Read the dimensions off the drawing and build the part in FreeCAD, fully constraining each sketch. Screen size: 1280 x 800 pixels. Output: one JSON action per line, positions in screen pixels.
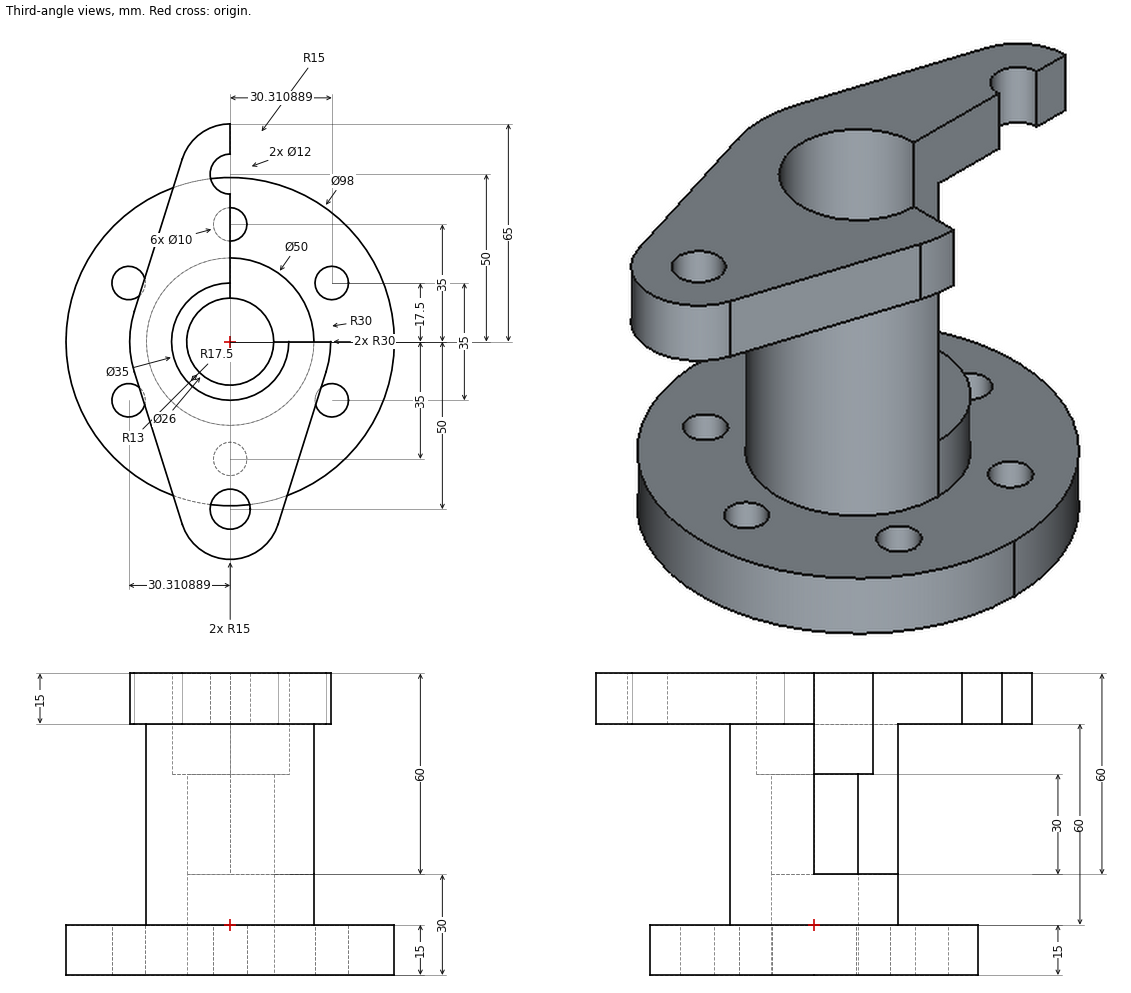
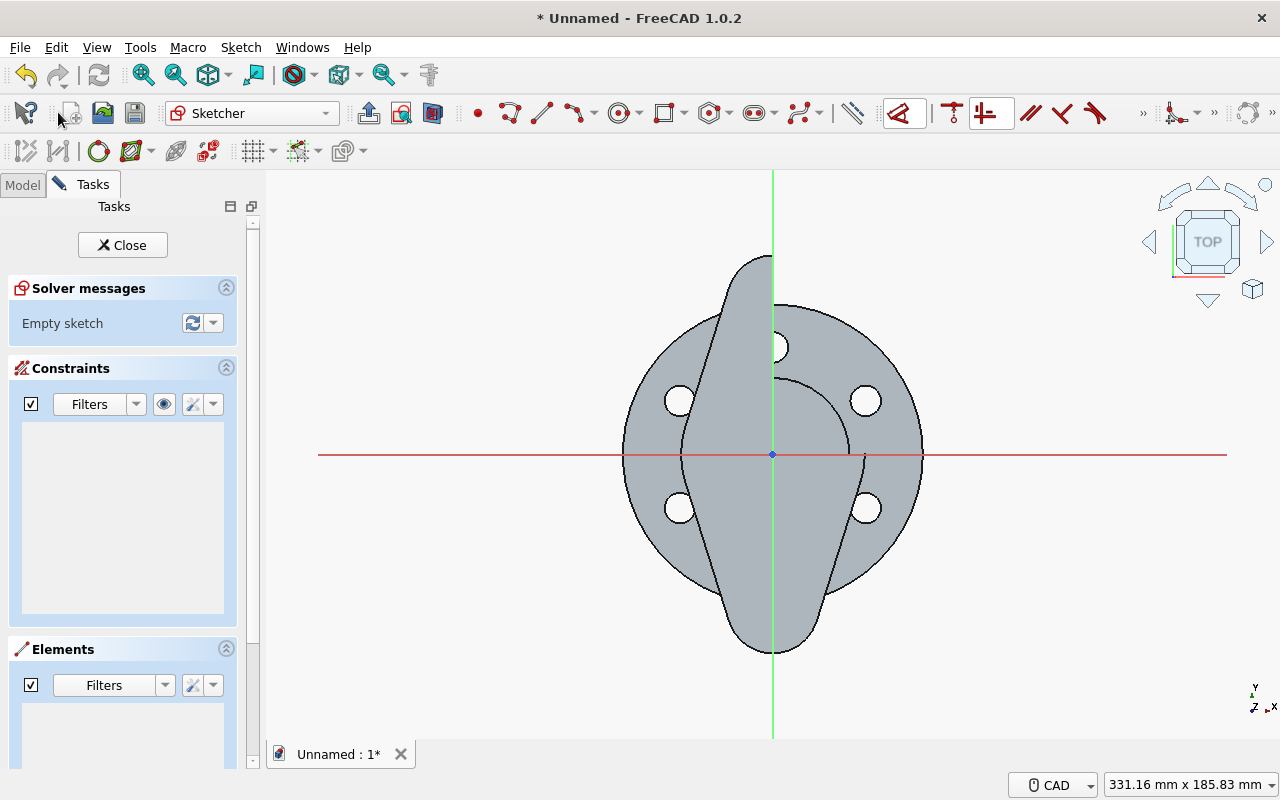
{"action": "key", "text": "g c"}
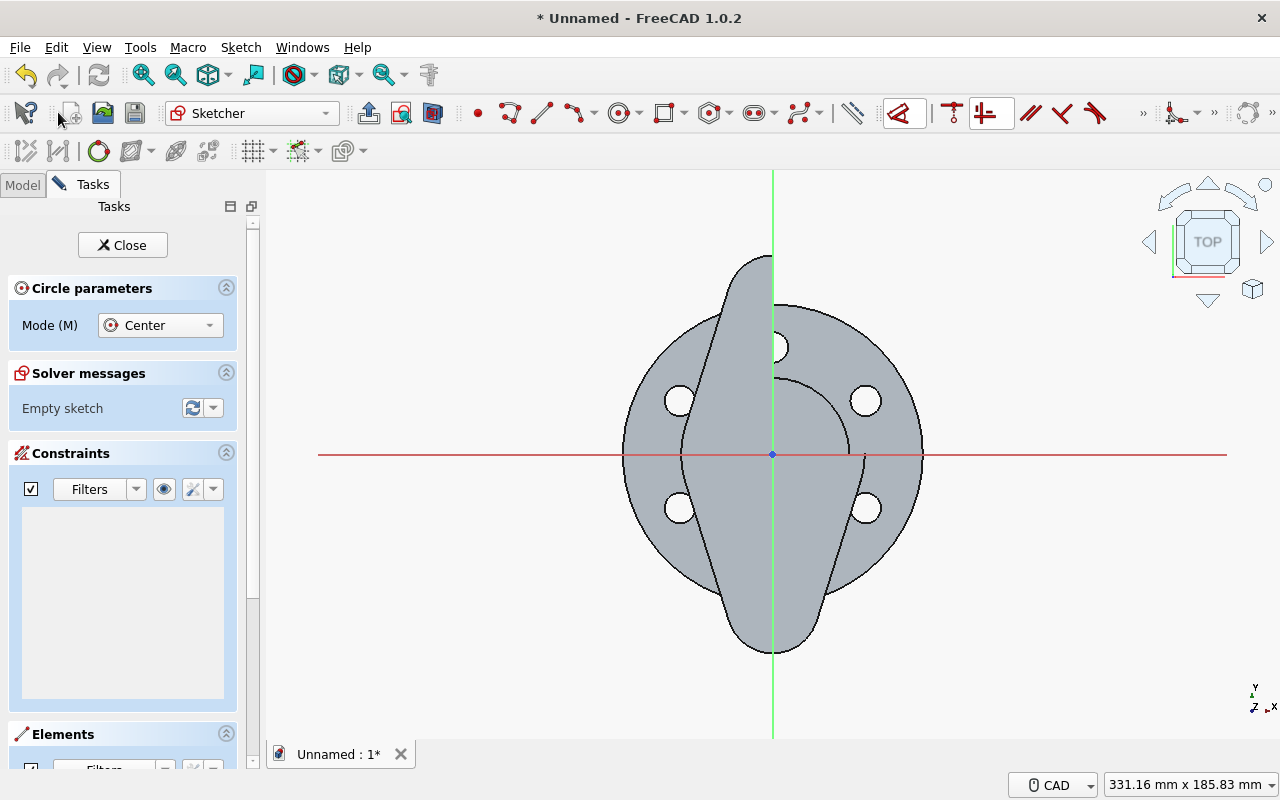
{"action": "left_click", "coordinate": [773, 454]}
{"action": "left_click", "coordinate": [811, 417]}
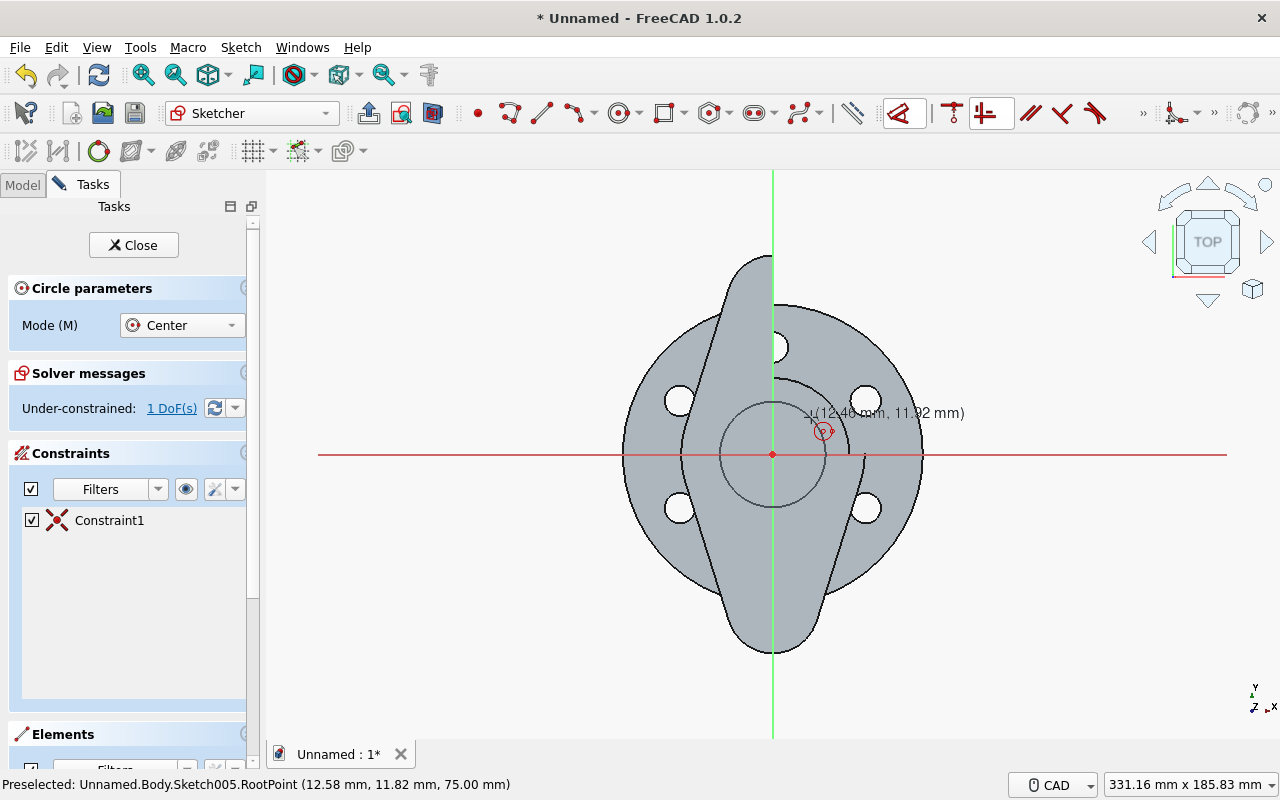
{"action": "scroll", "coordinate": [773, 301], "scroll_direction": "up", "scroll_amount": 2}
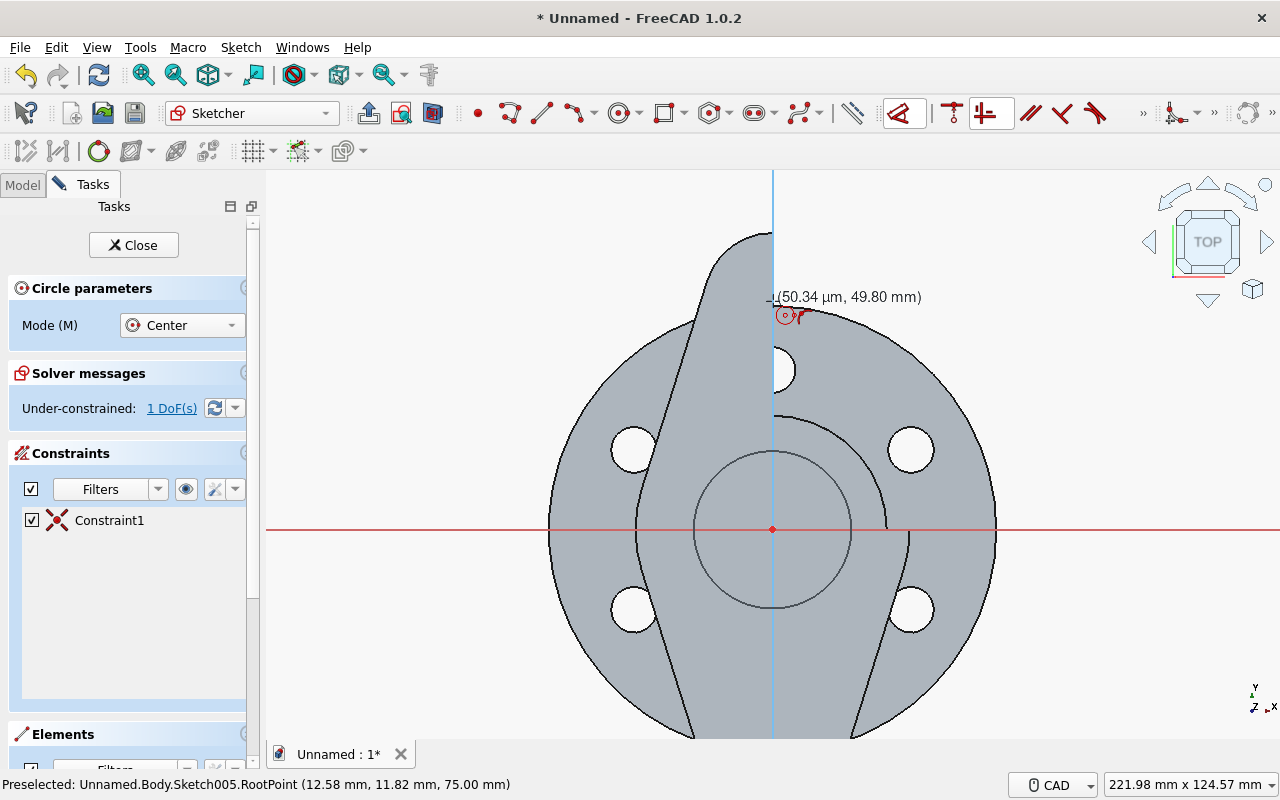
{"action": "left_click", "coordinate": [773, 301]}
{"action": "left_click", "coordinate": [792, 282]}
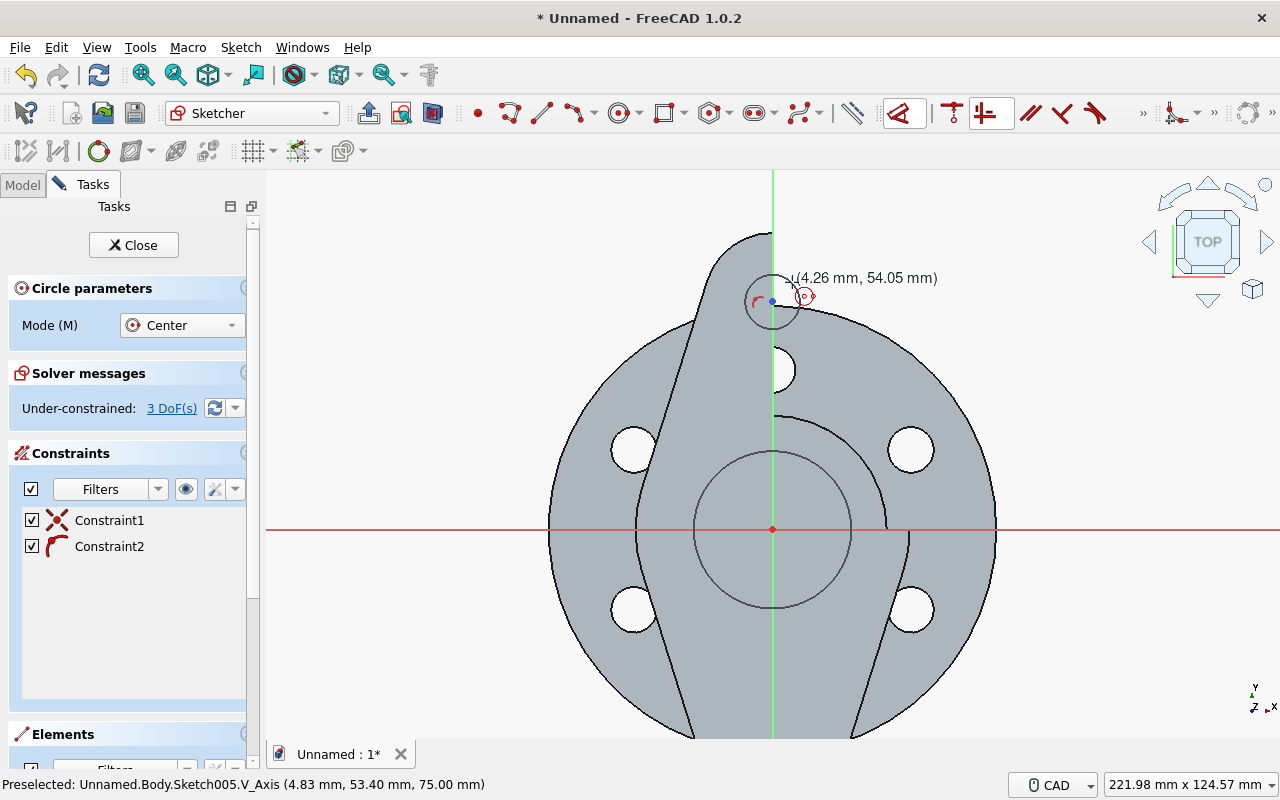
{"action": "scroll", "coordinate": [566, 301], "scroll_direction": "down", "scroll_amount": 2}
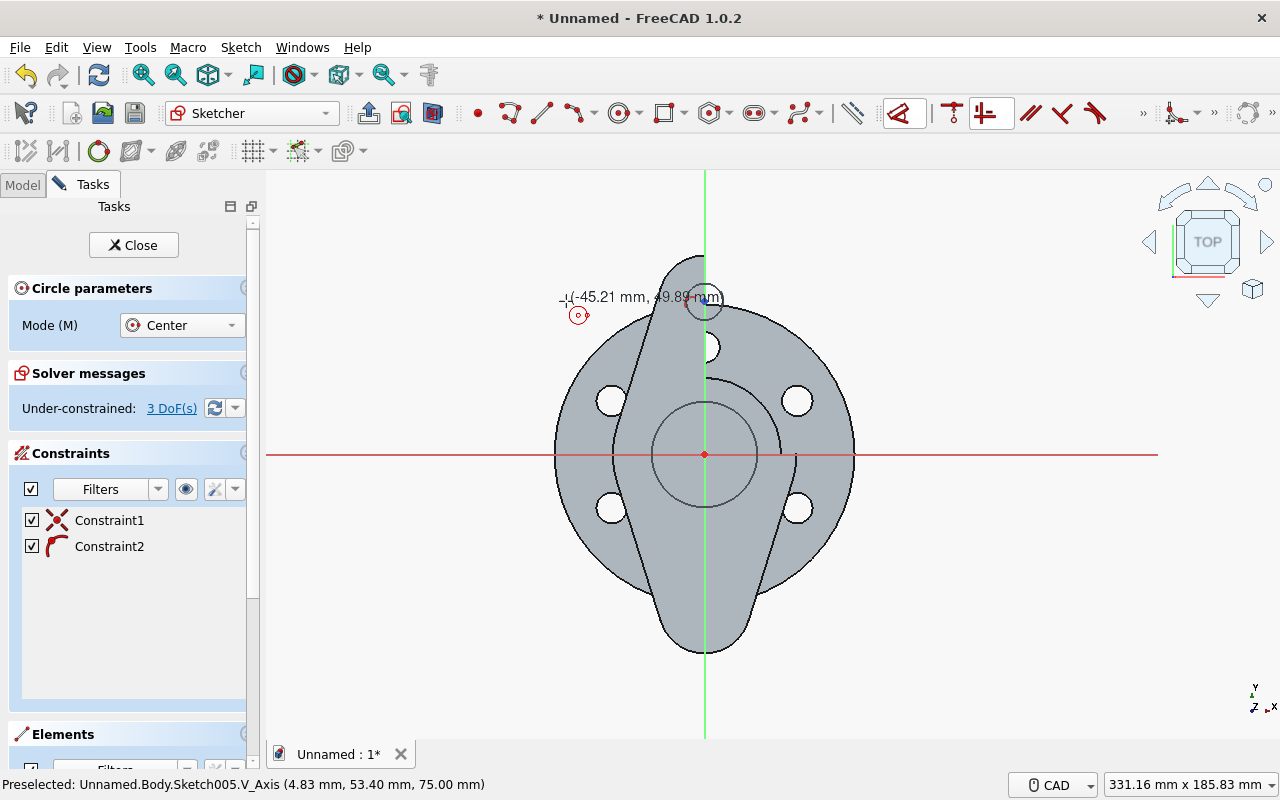
{"action": "scroll", "coordinate": [705, 608], "scroll_direction": "up", "scroll_amount": 2}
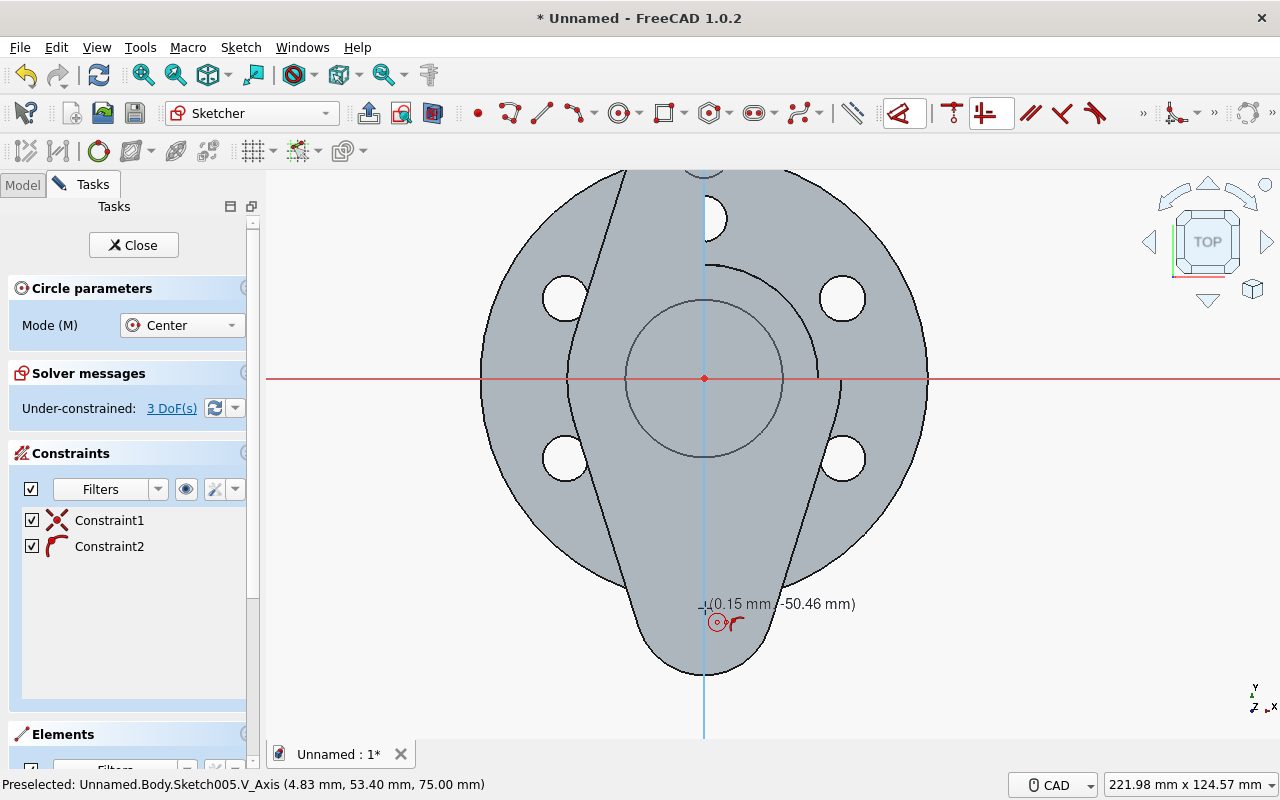
{"action": "left_click", "coordinate": [704, 607]}
{"action": "left_click", "coordinate": [723, 588]}
{"action": "key", "text": "Escape"}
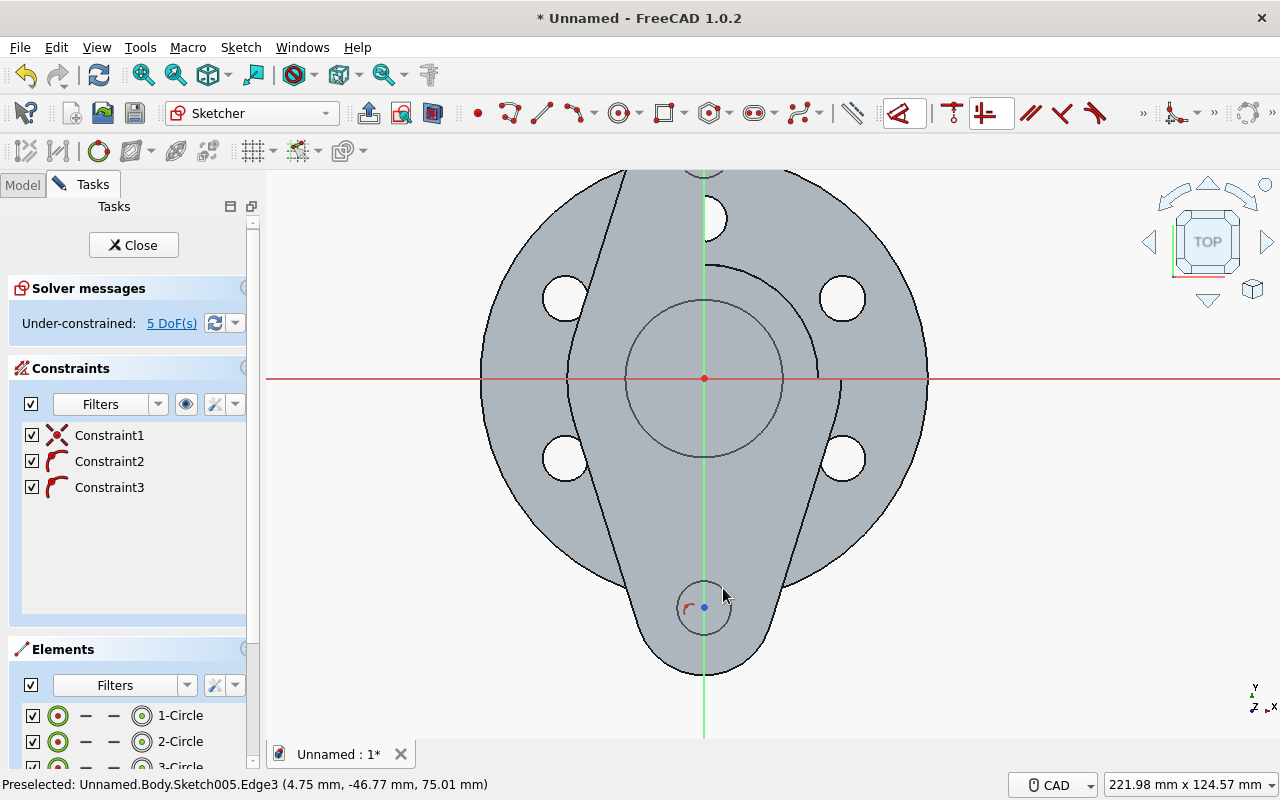
{"action": "scroll", "coordinate": [705, 609], "scroll_direction": "down", "scroll_amount": 2}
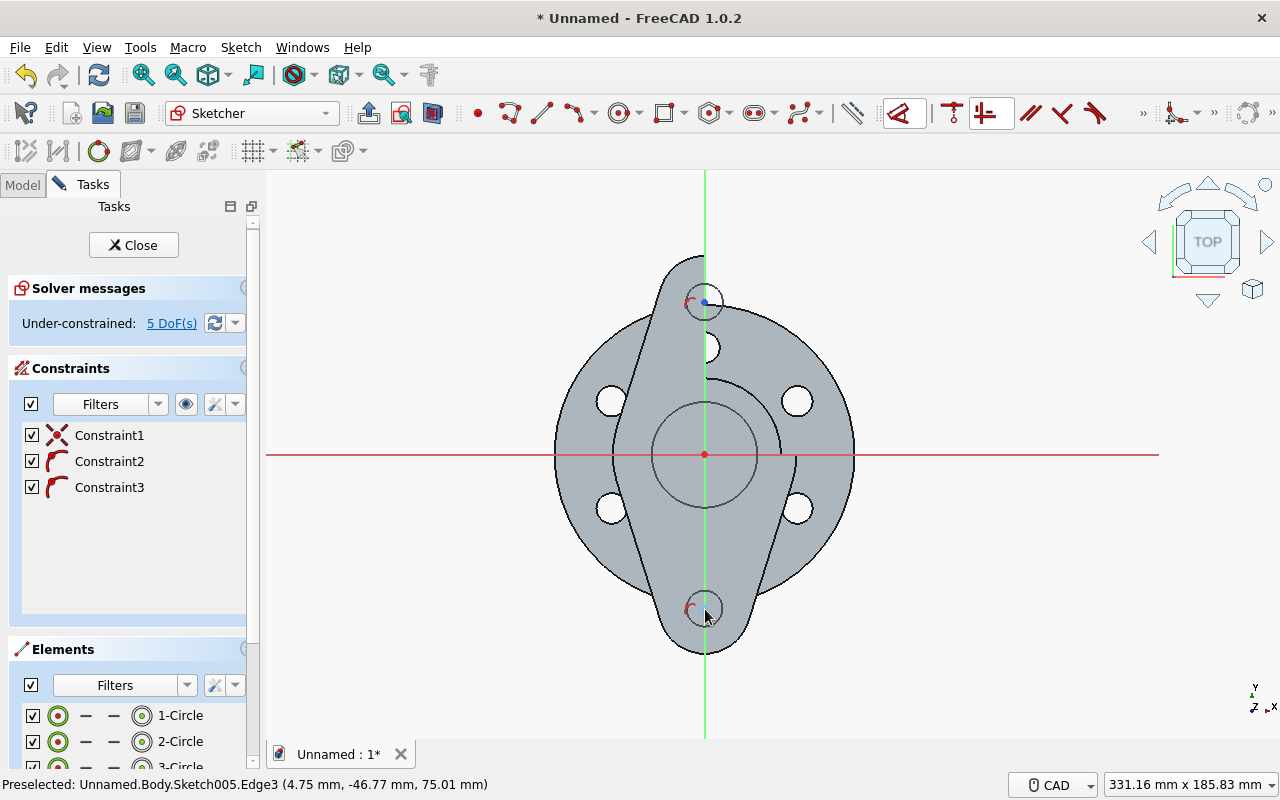
{"action": "left_click", "coordinate": [717, 289]}